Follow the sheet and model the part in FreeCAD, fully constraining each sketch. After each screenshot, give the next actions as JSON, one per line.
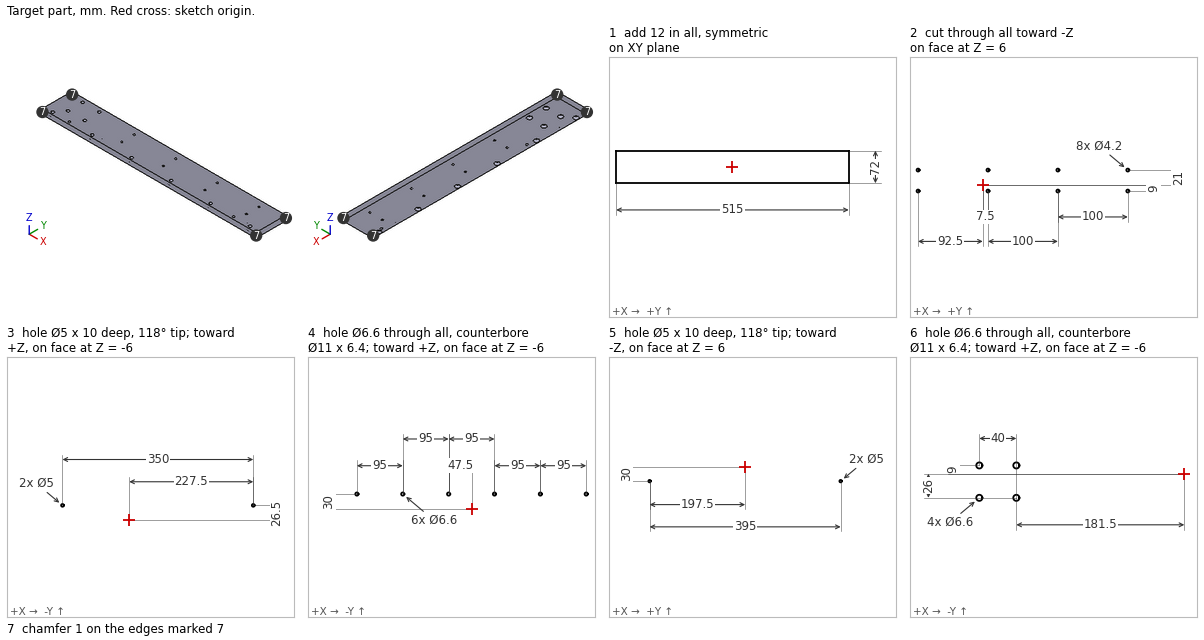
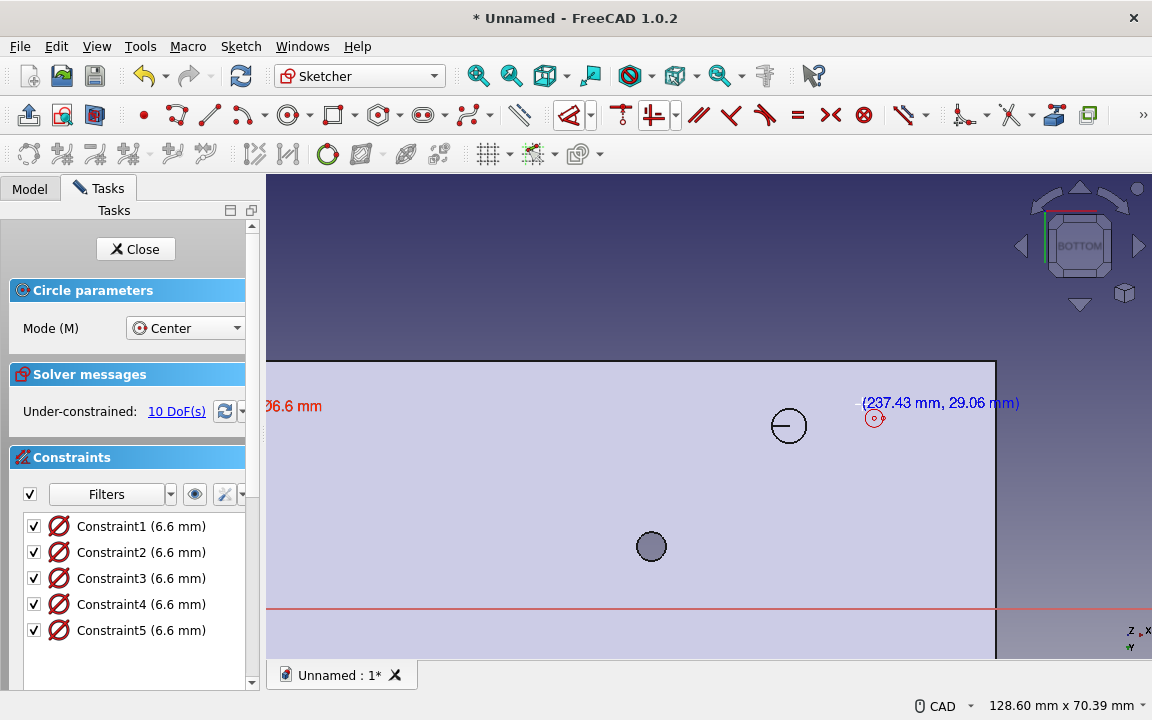
{"action": "scroll", "coordinate": [863, 404], "scroll_direction": "down", "scroll_amount": 10}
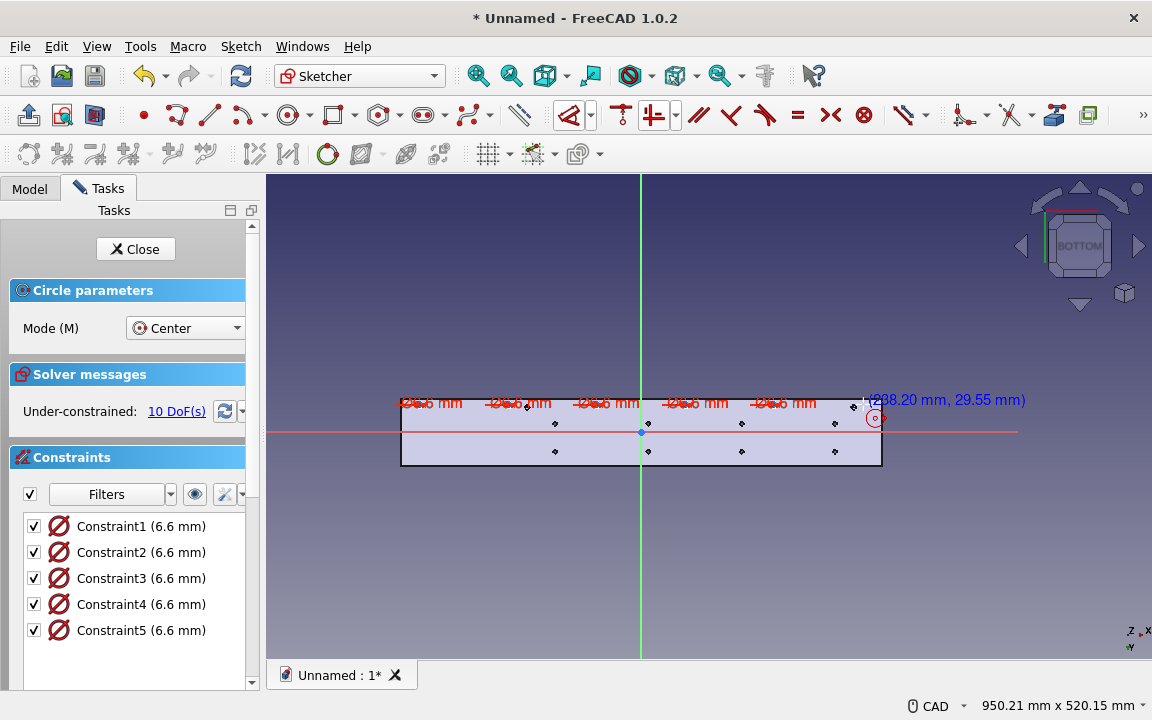
{"action": "left_click", "coordinate": [863, 404]}
{"action": "mouse_move", "coordinate": [865, 402]}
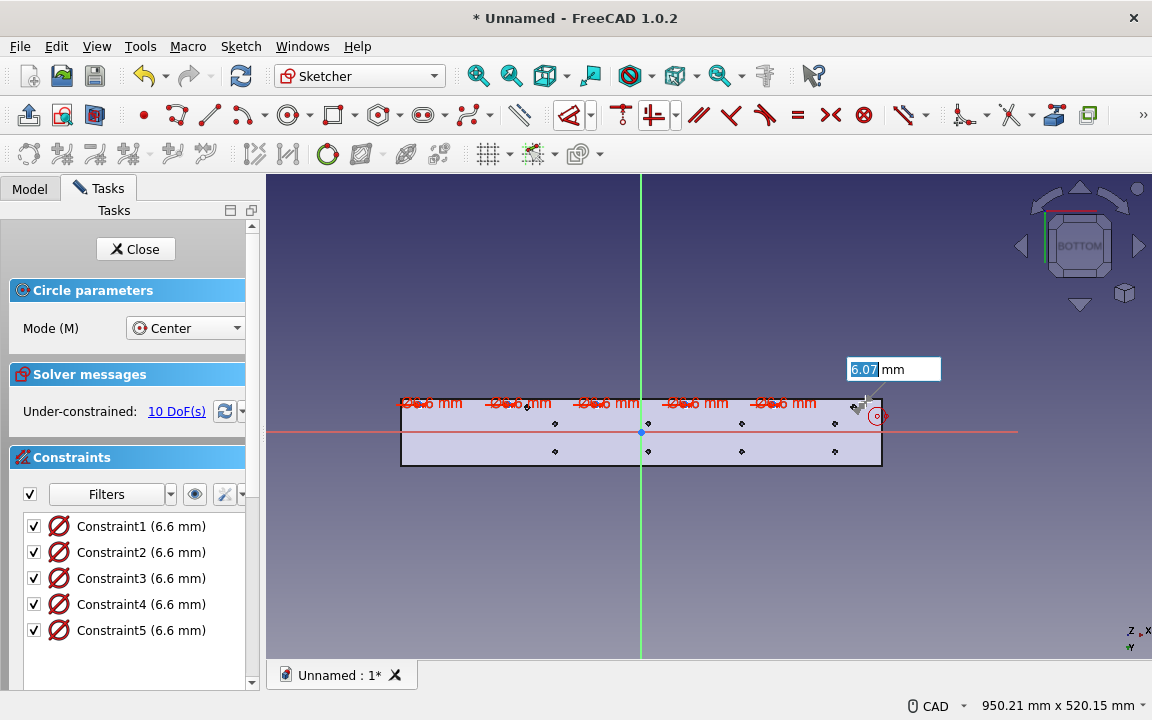
{"action": "type", "text": "6.6"}
{"action": "key", "text": "Return"}
{"action": "key", "text": "Escape"}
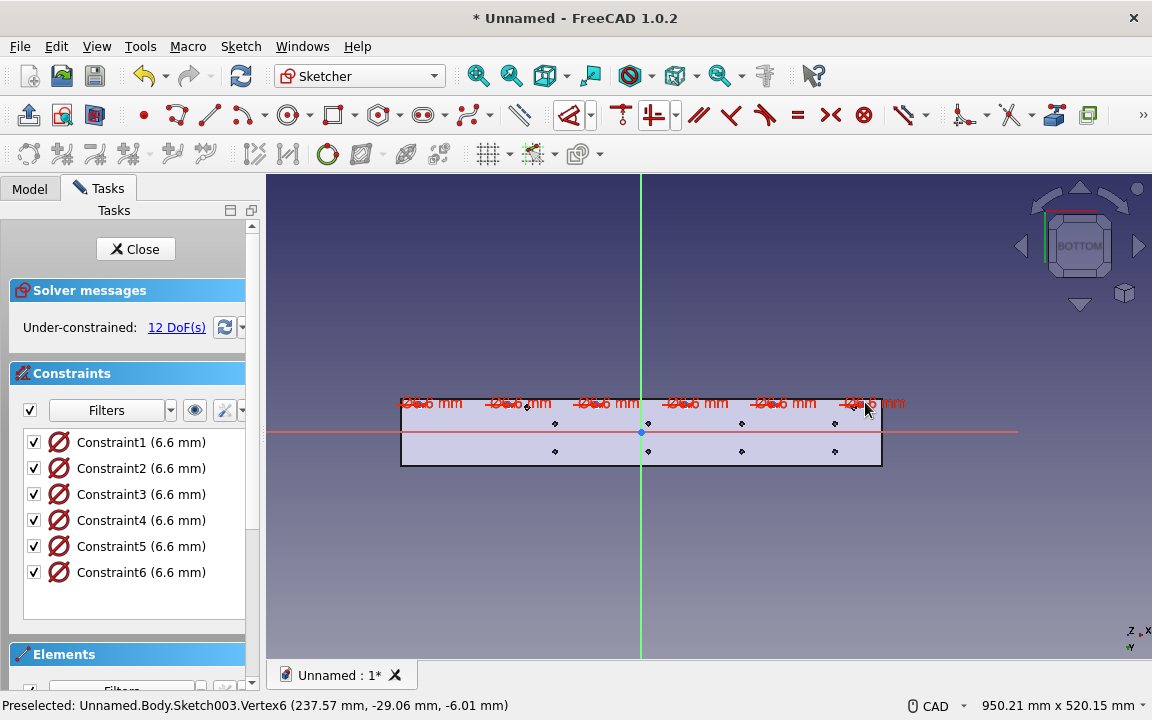
{"action": "left_click", "coordinate": [420, 405]}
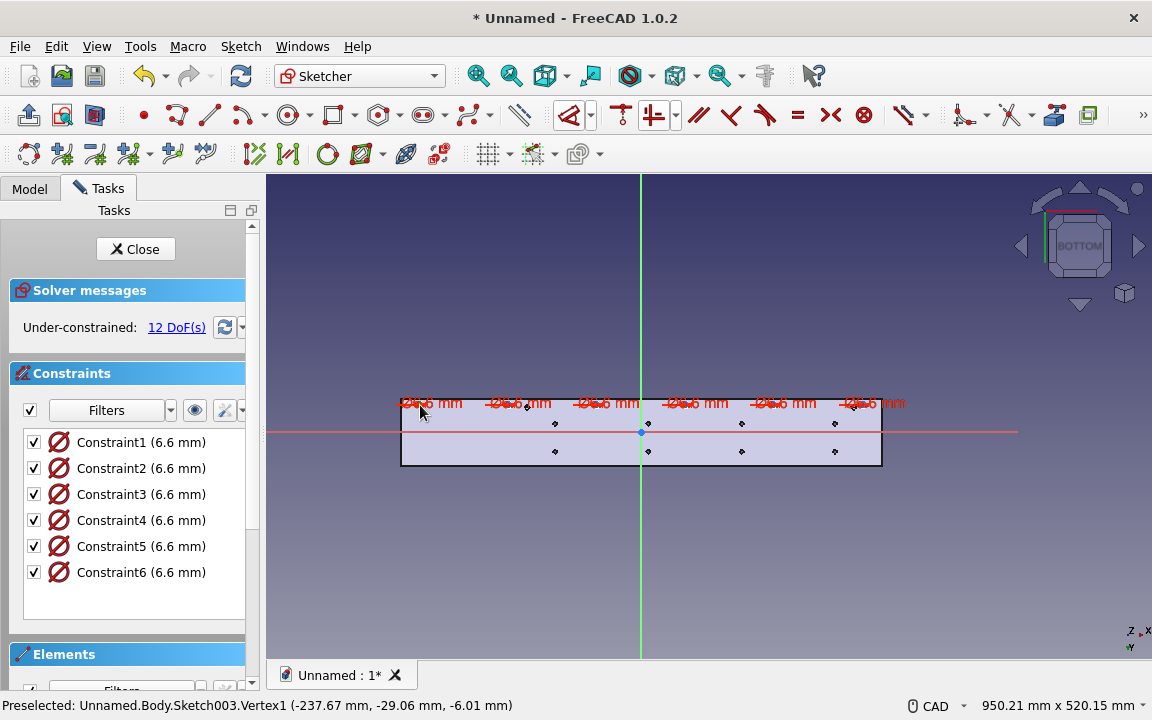
{"action": "left_click", "coordinate": [509, 405]}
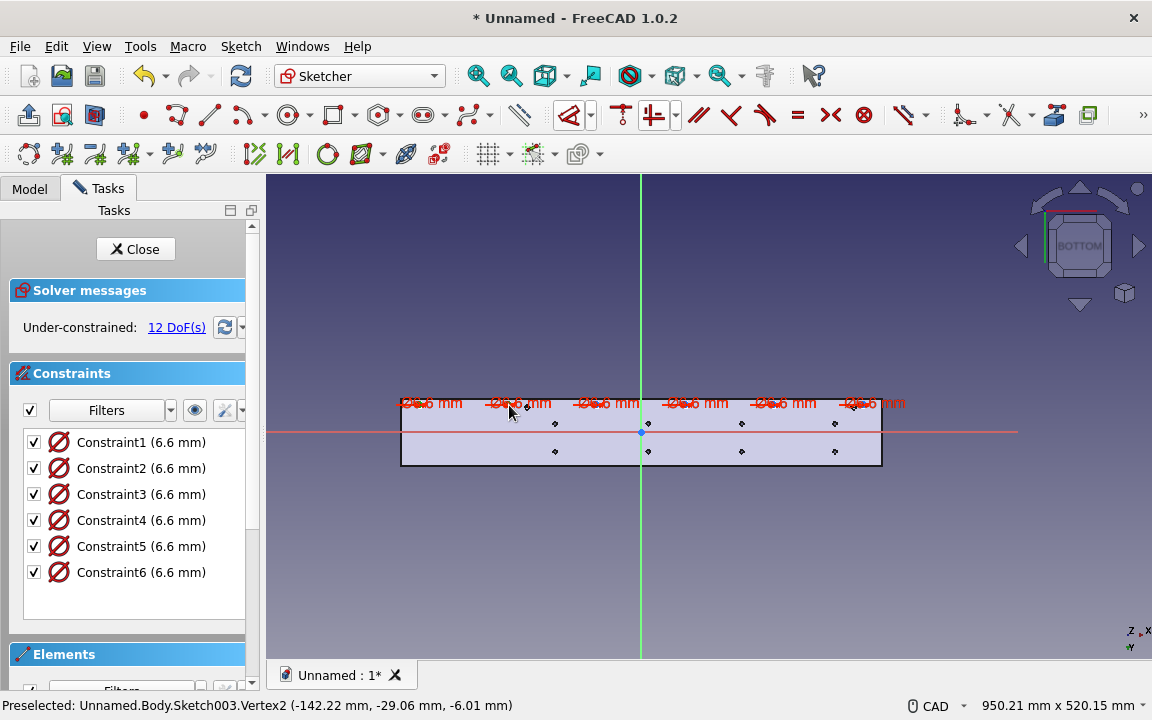
{"action": "left_click", "coordinate": [676, 116]}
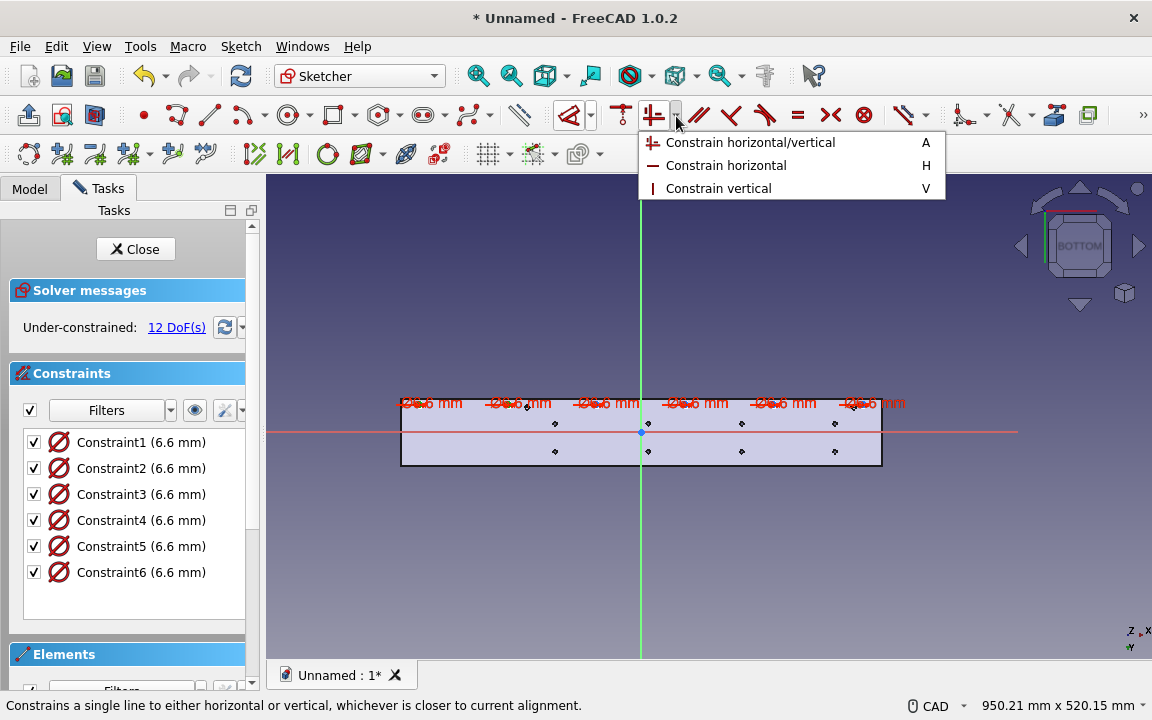
{"action": "left_click", "coordinate": [792, 166]}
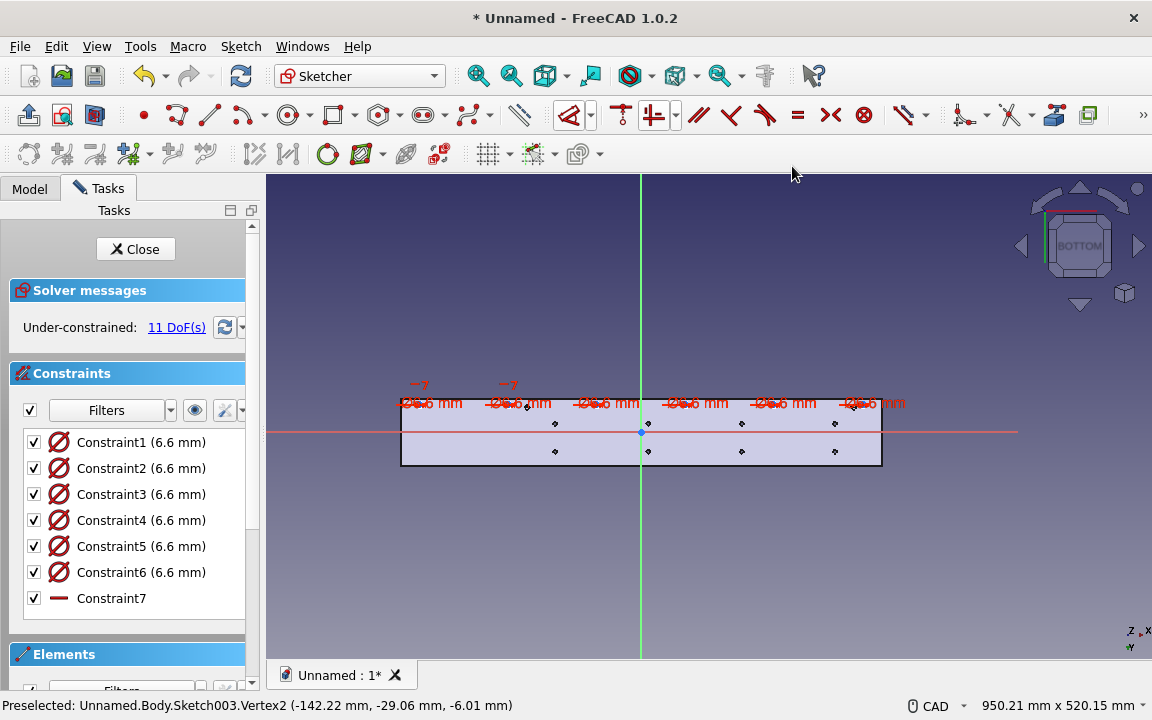
{"action": "left_click", "coordinate": [509, 405]}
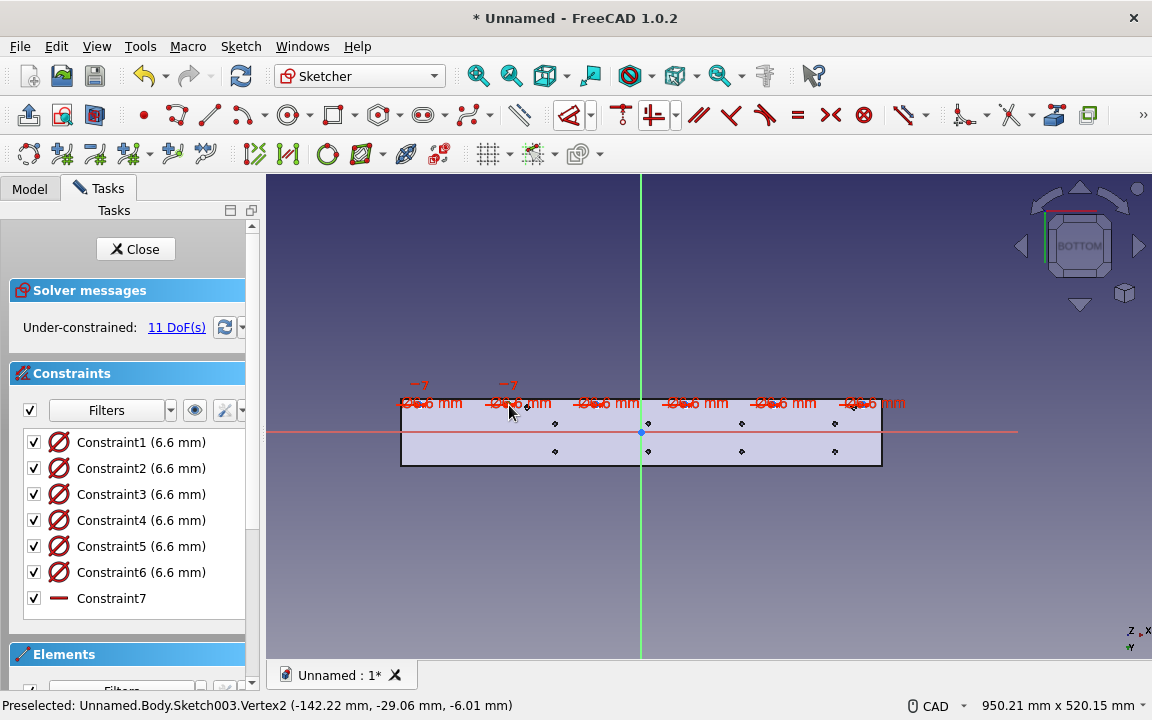
{"action": "left_click", "coordinate": [597, 405]}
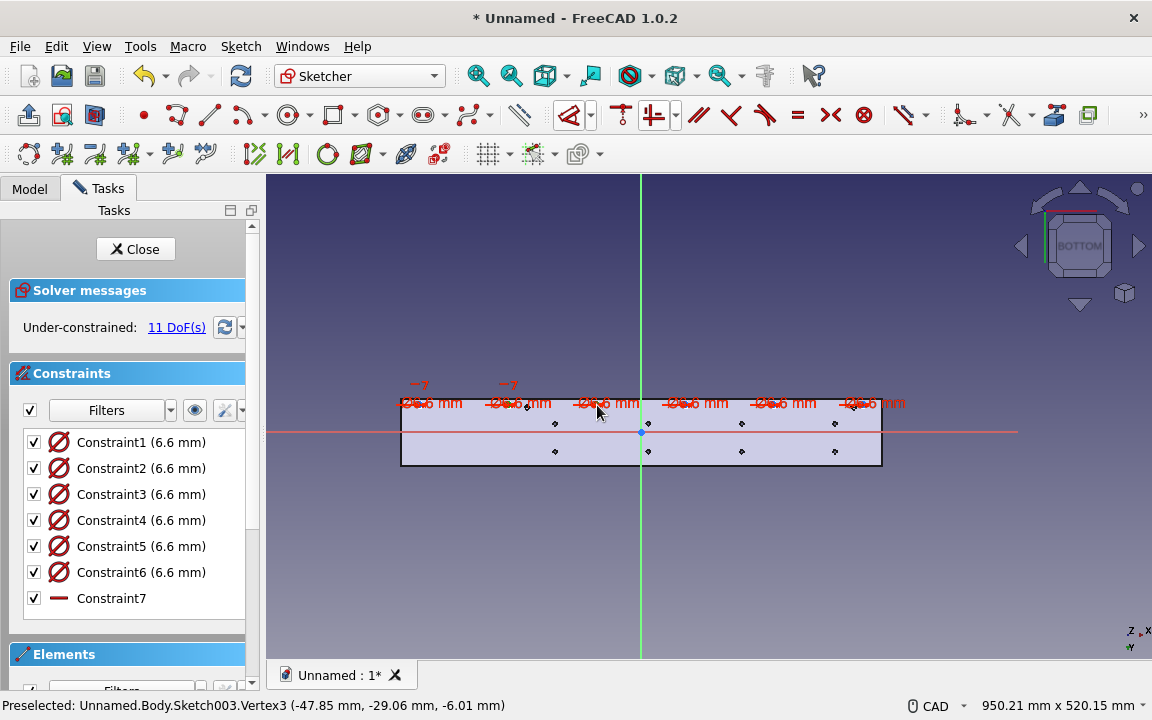
{"action": "key", "text": "h"}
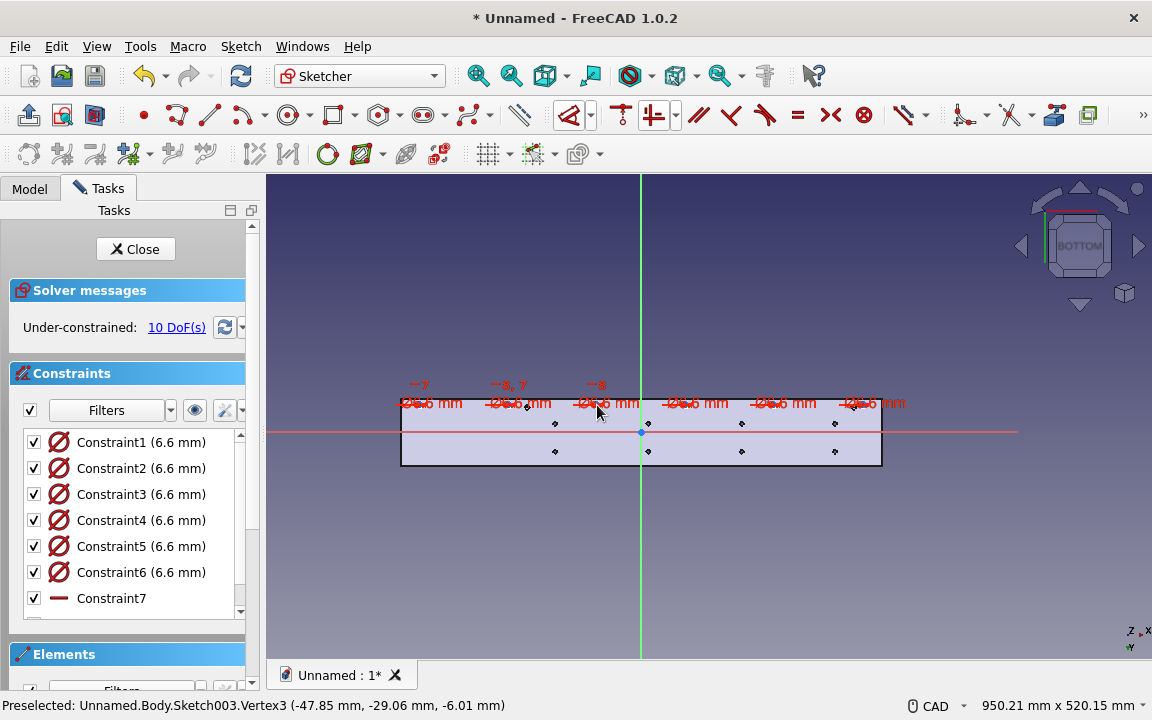
{"action": "left_click", "coordinate": [597, 405]}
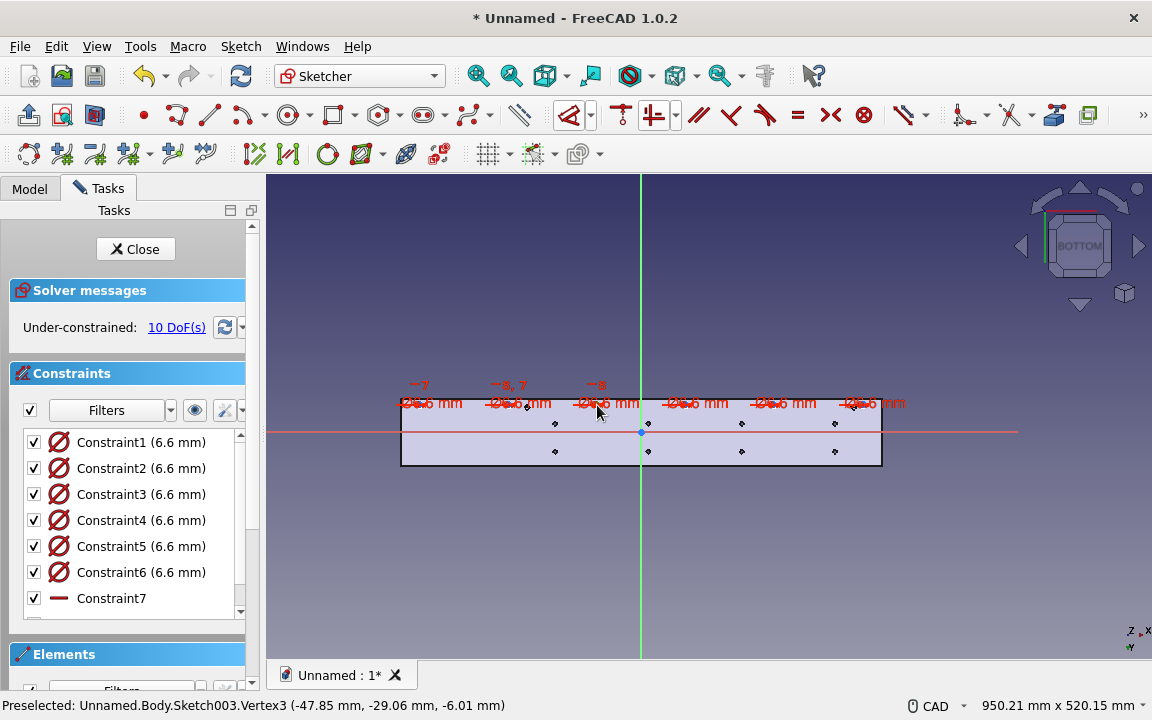
{"action": "left_click", "coordinate": [686, 405]}